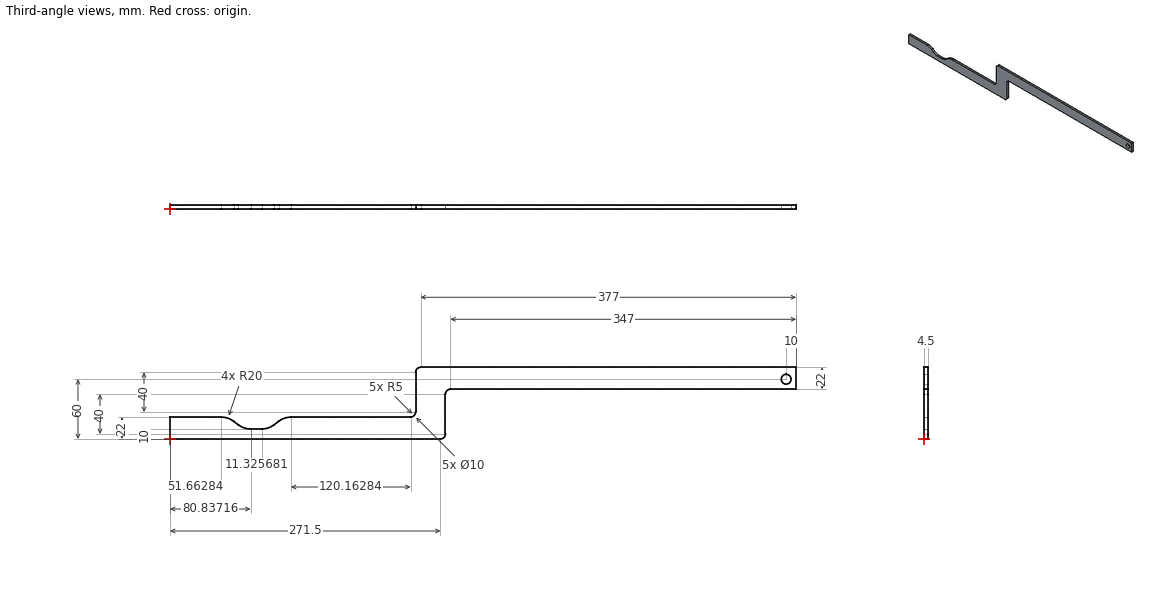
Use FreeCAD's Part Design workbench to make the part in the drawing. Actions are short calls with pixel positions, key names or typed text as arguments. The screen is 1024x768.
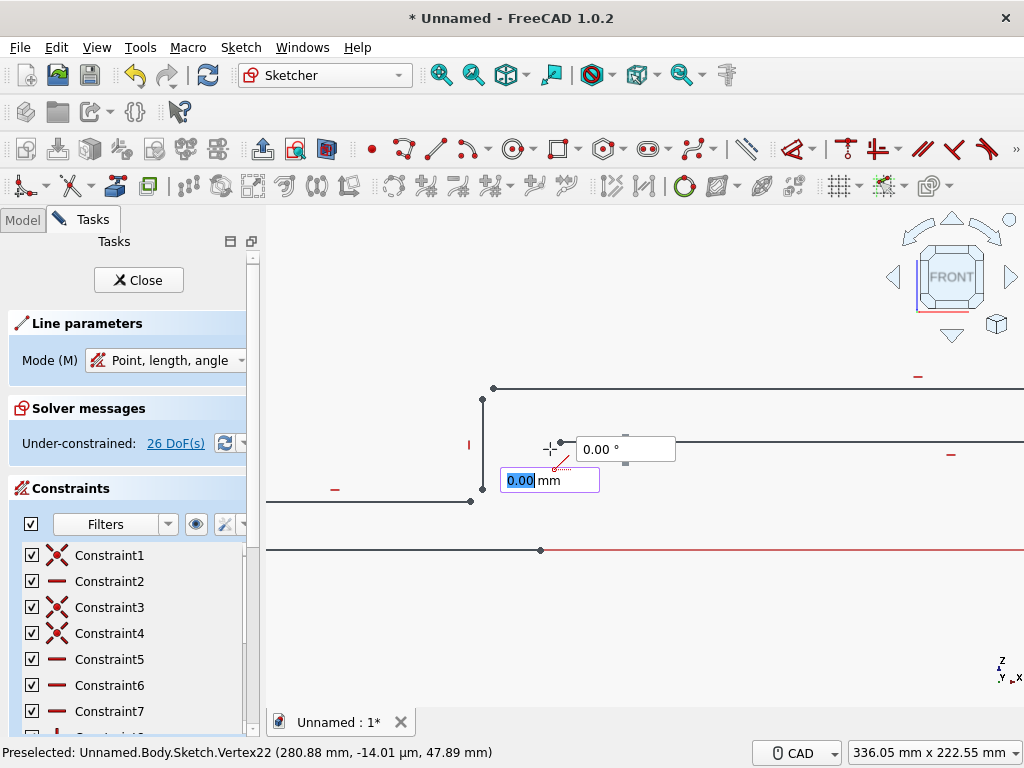
scroll(550, 539, up, 2)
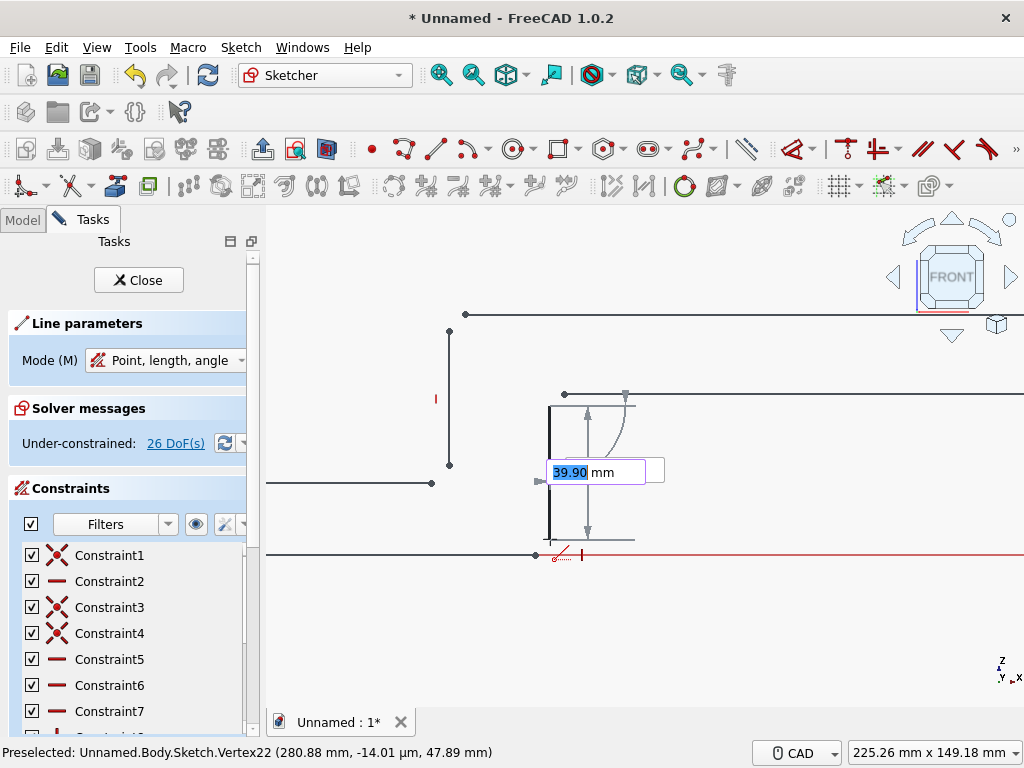
click(550, 539)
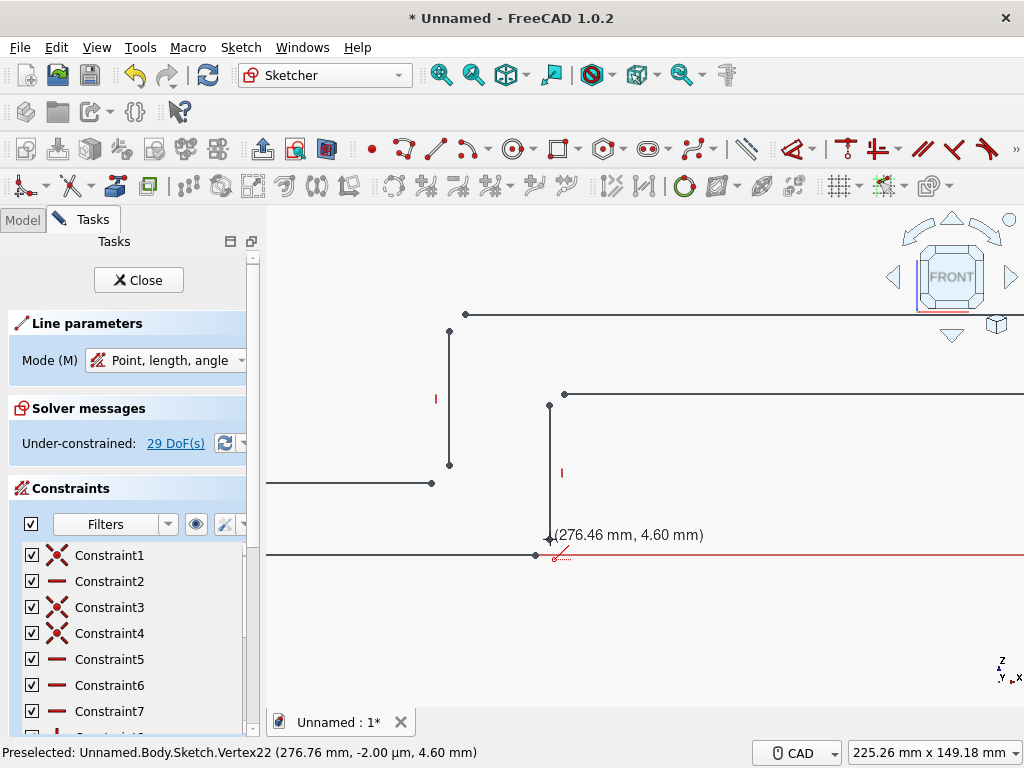
key(g)
key(3)
key(a)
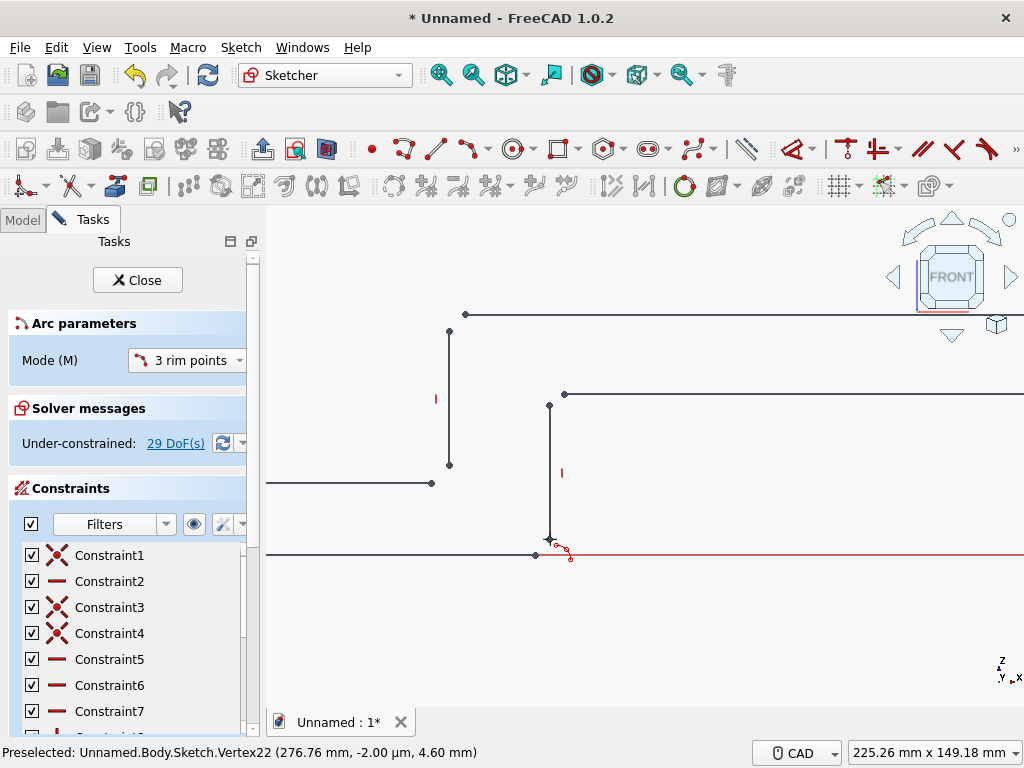
scroll(551, 461, down, 8)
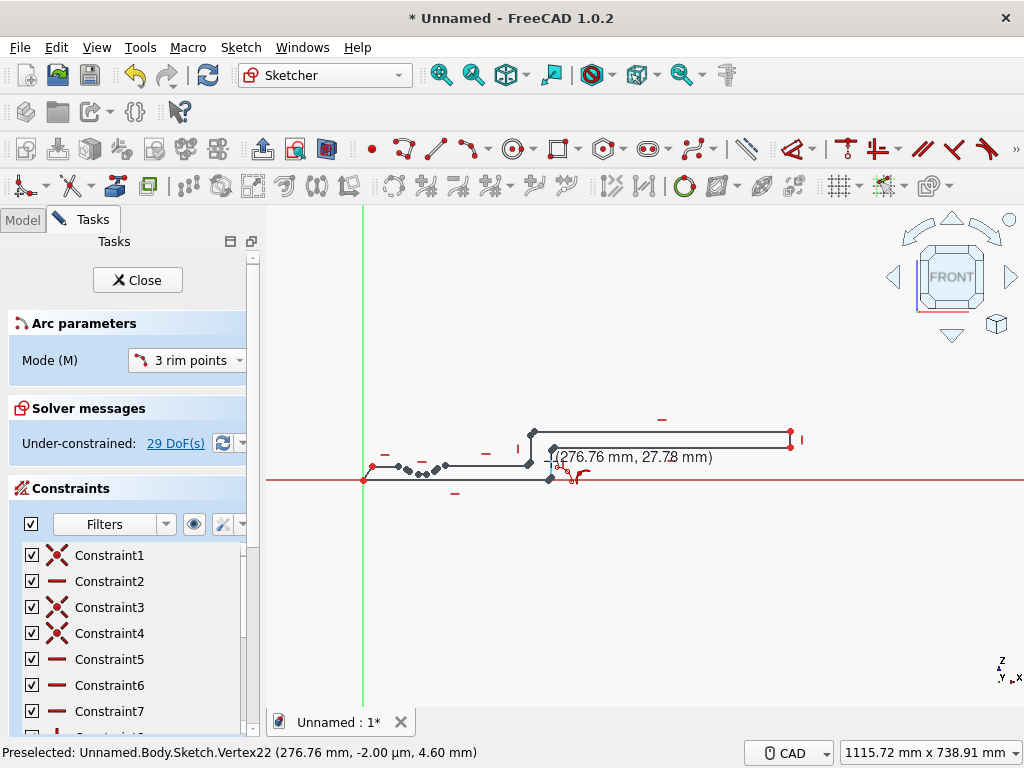
scroll(398, 466, up, 3)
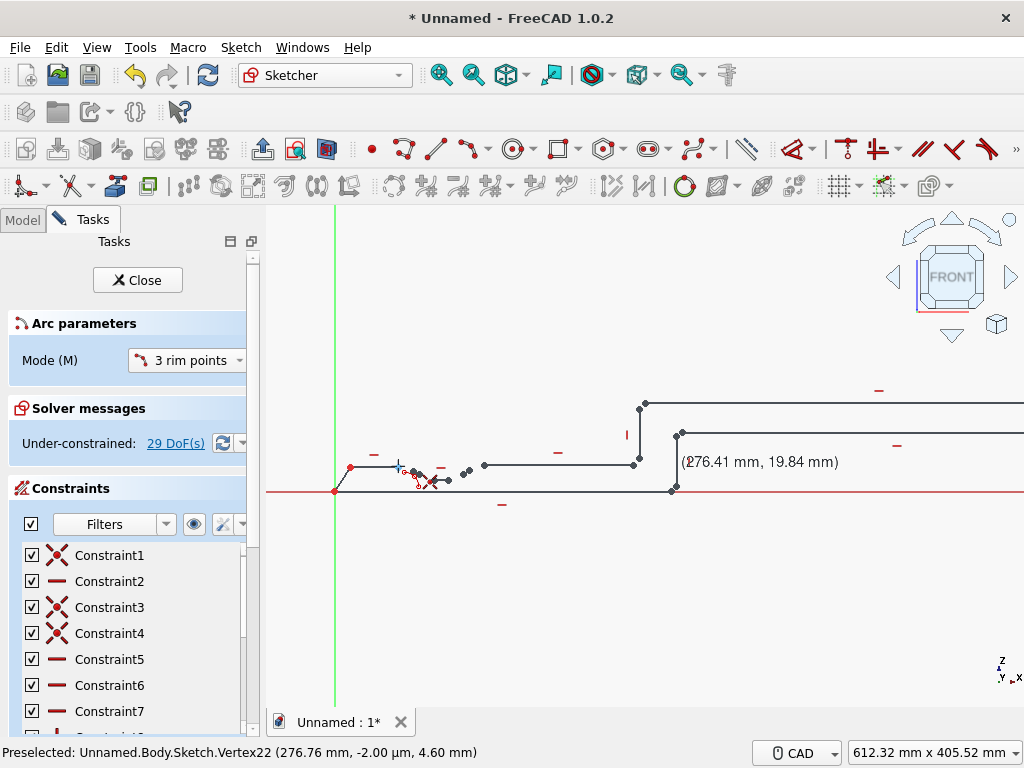
click(398, 467)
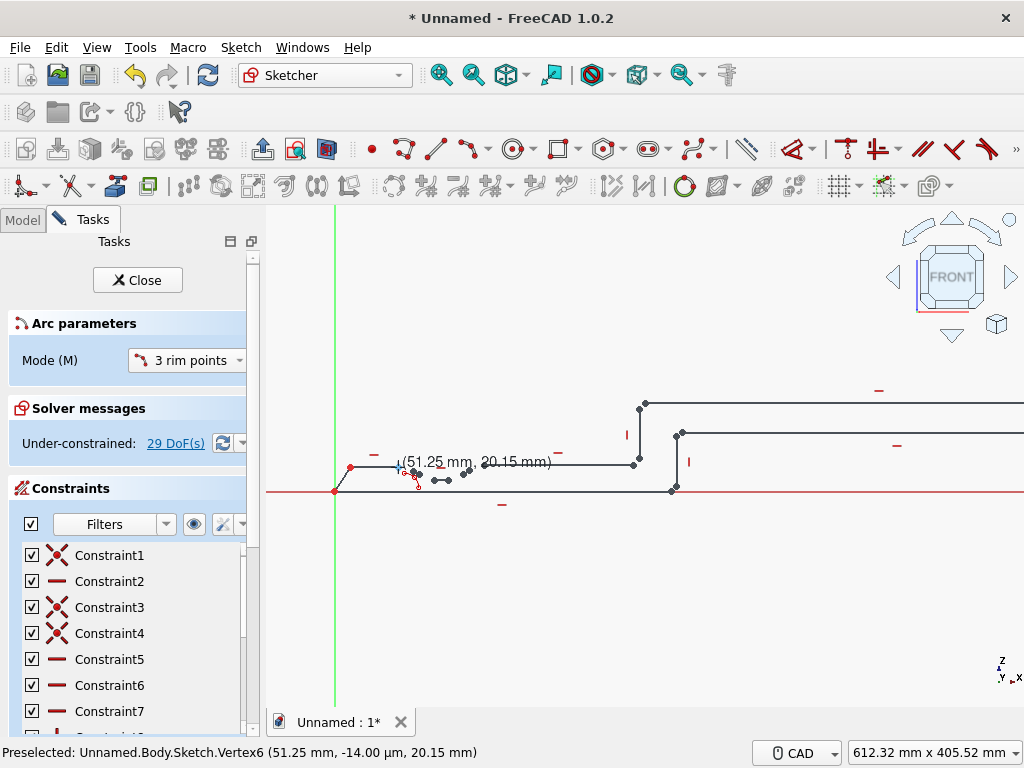
scroll(414, 470, up, 8)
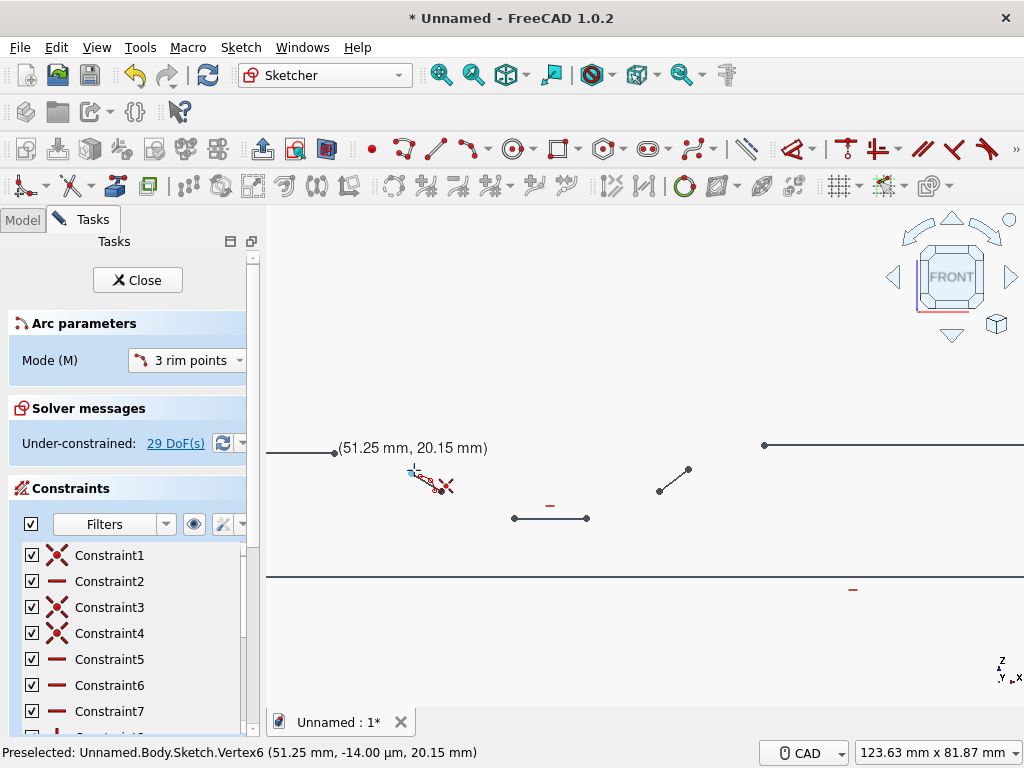
click(411, 473)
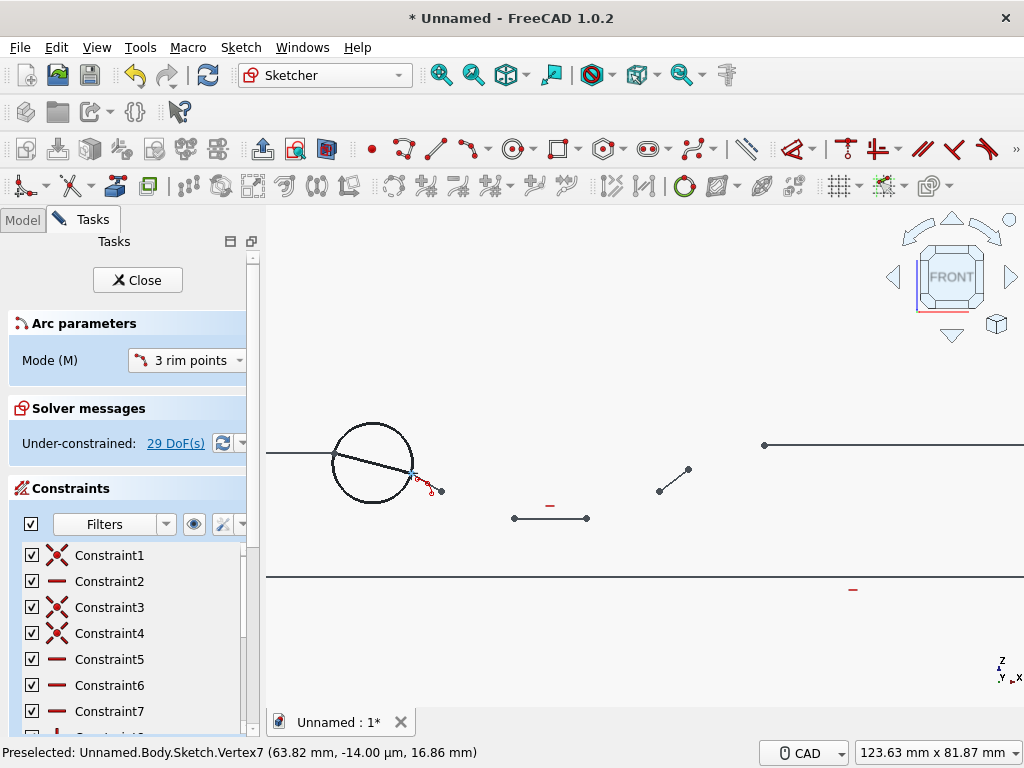
scroll(376, 448, up, 5)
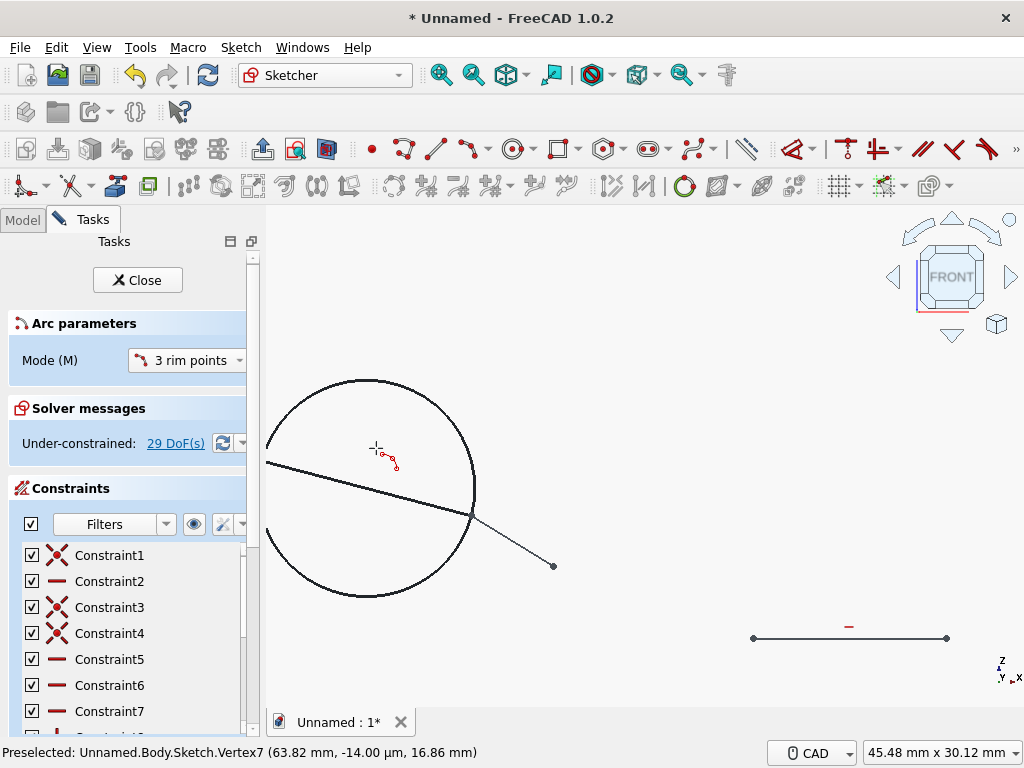
click(377, 448)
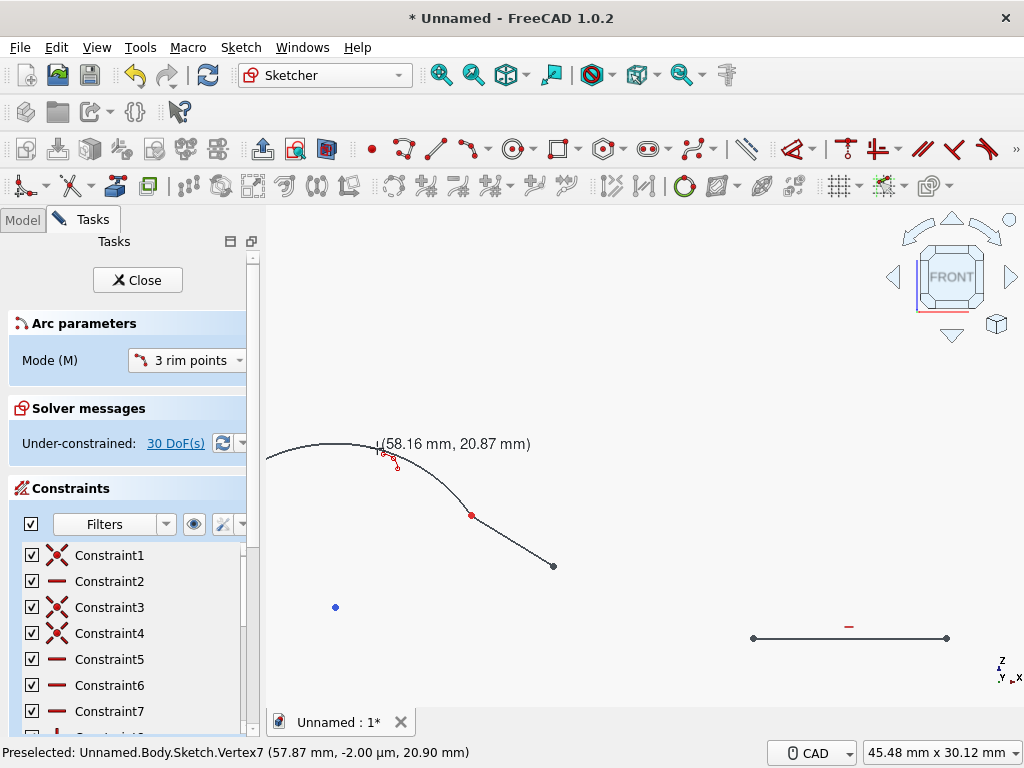
scroll(404, 467, down, 16)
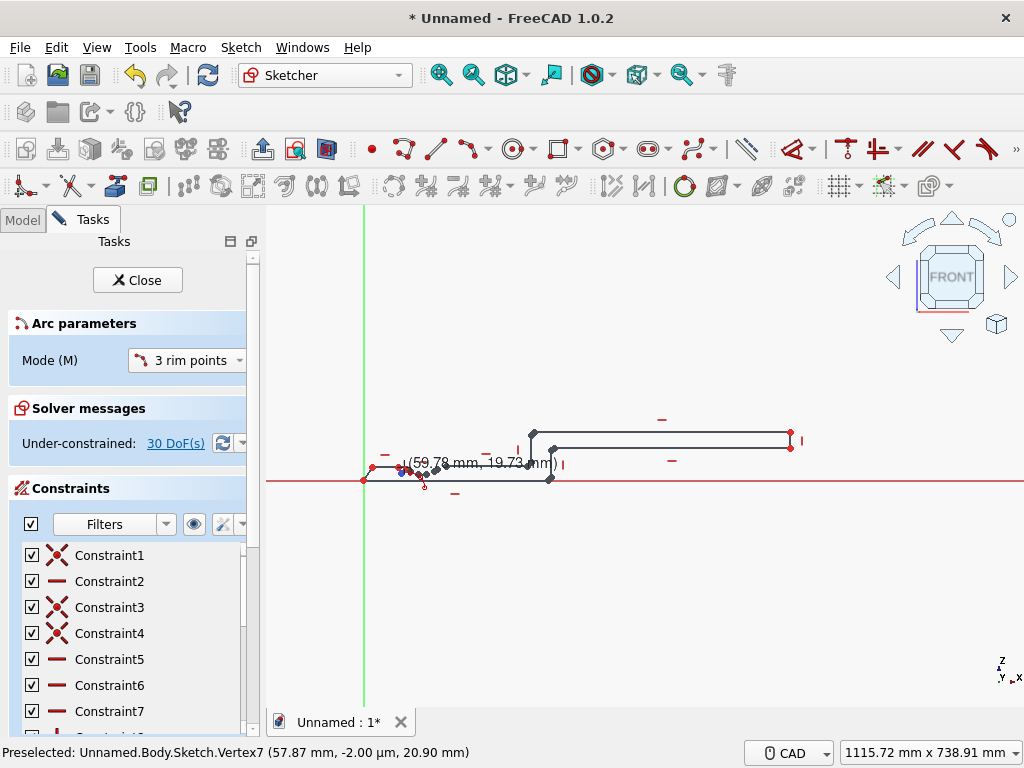
scroll(410, 471, up, 11)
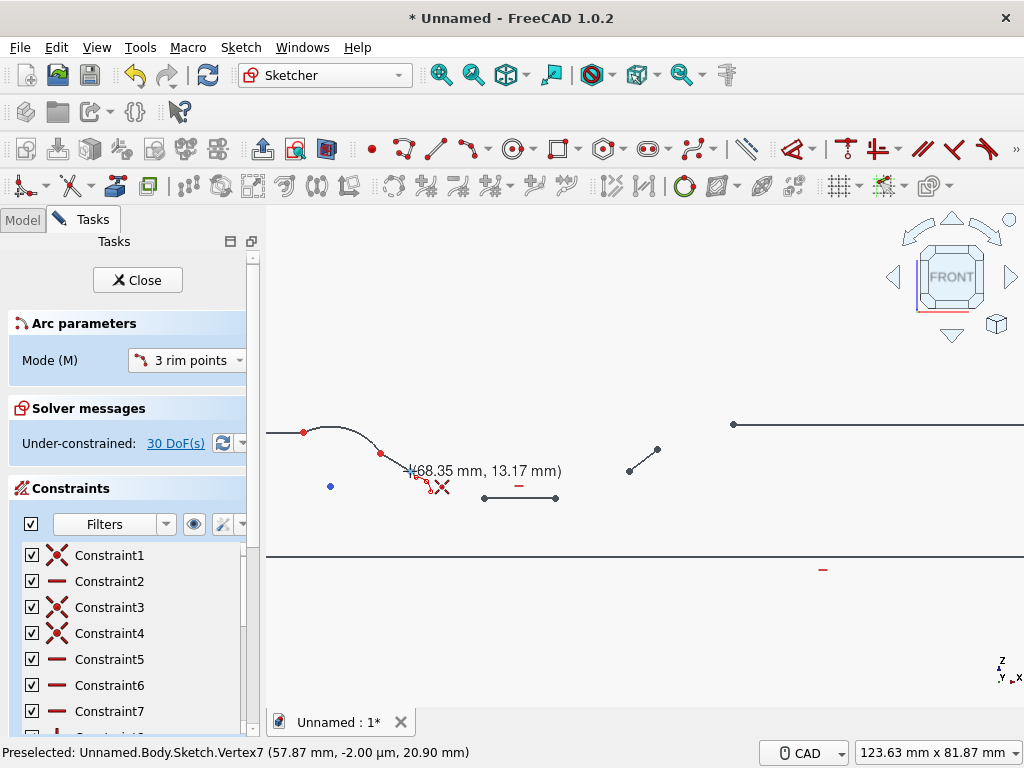
click(411, 472)
click(484, 498)